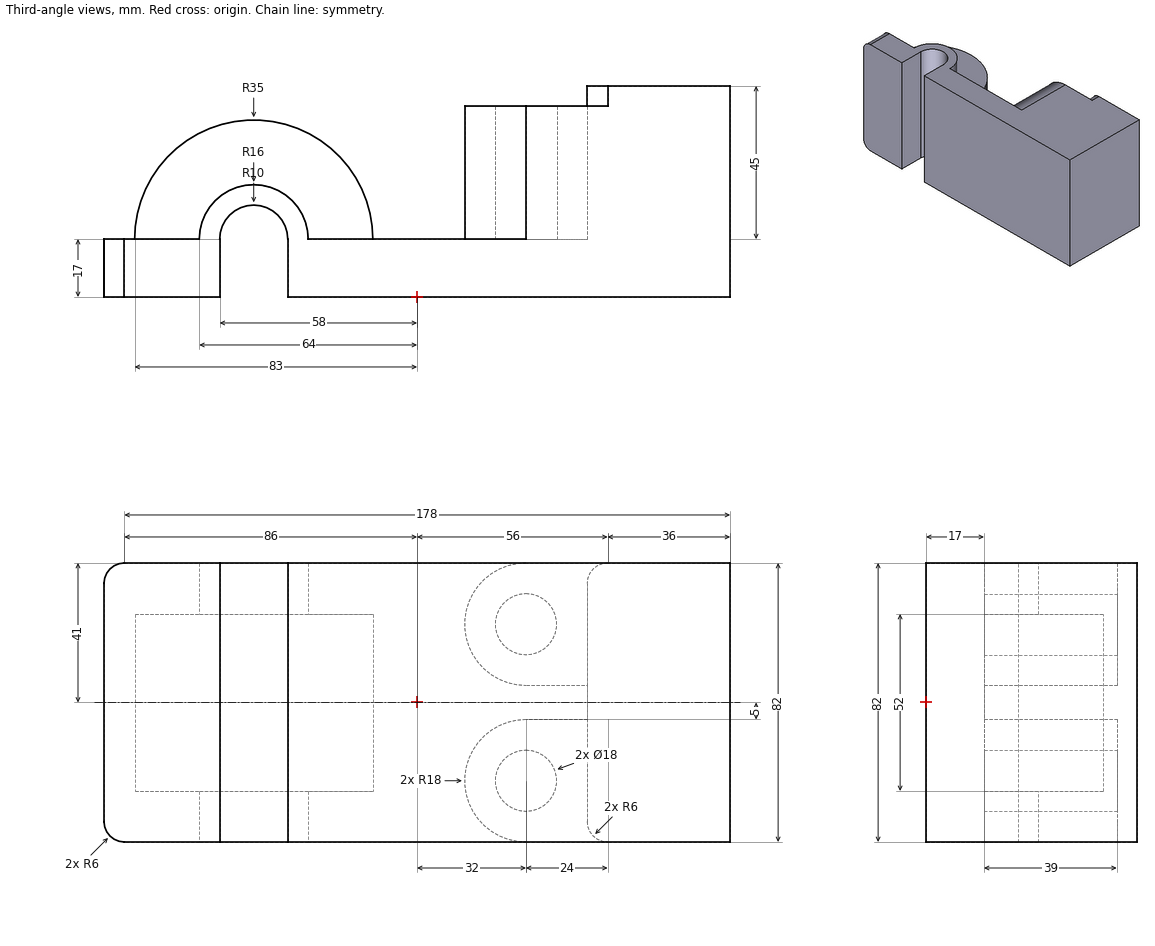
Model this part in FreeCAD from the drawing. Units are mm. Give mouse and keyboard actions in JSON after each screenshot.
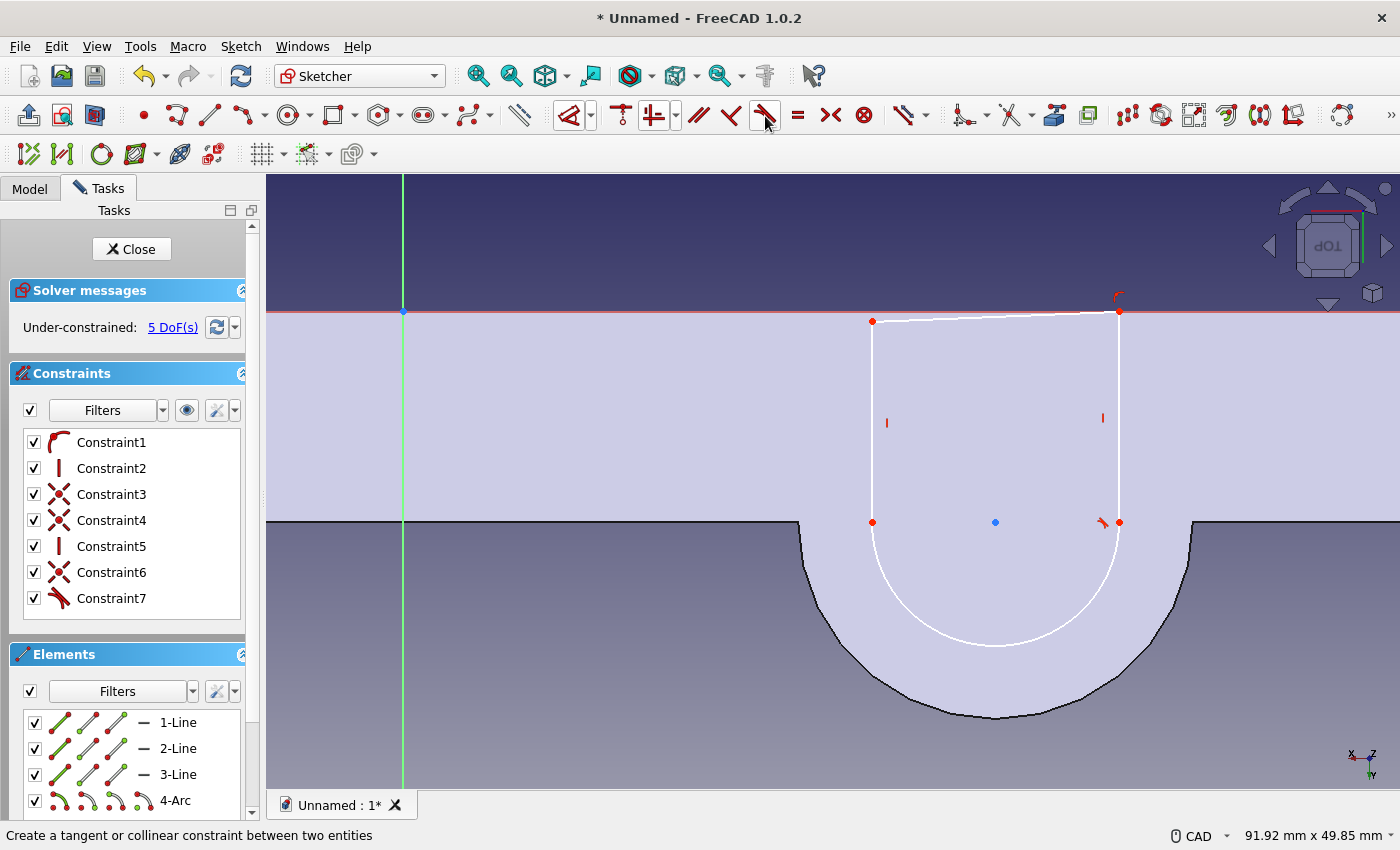
{"action": "left_click", "coordinate": [872, 382]}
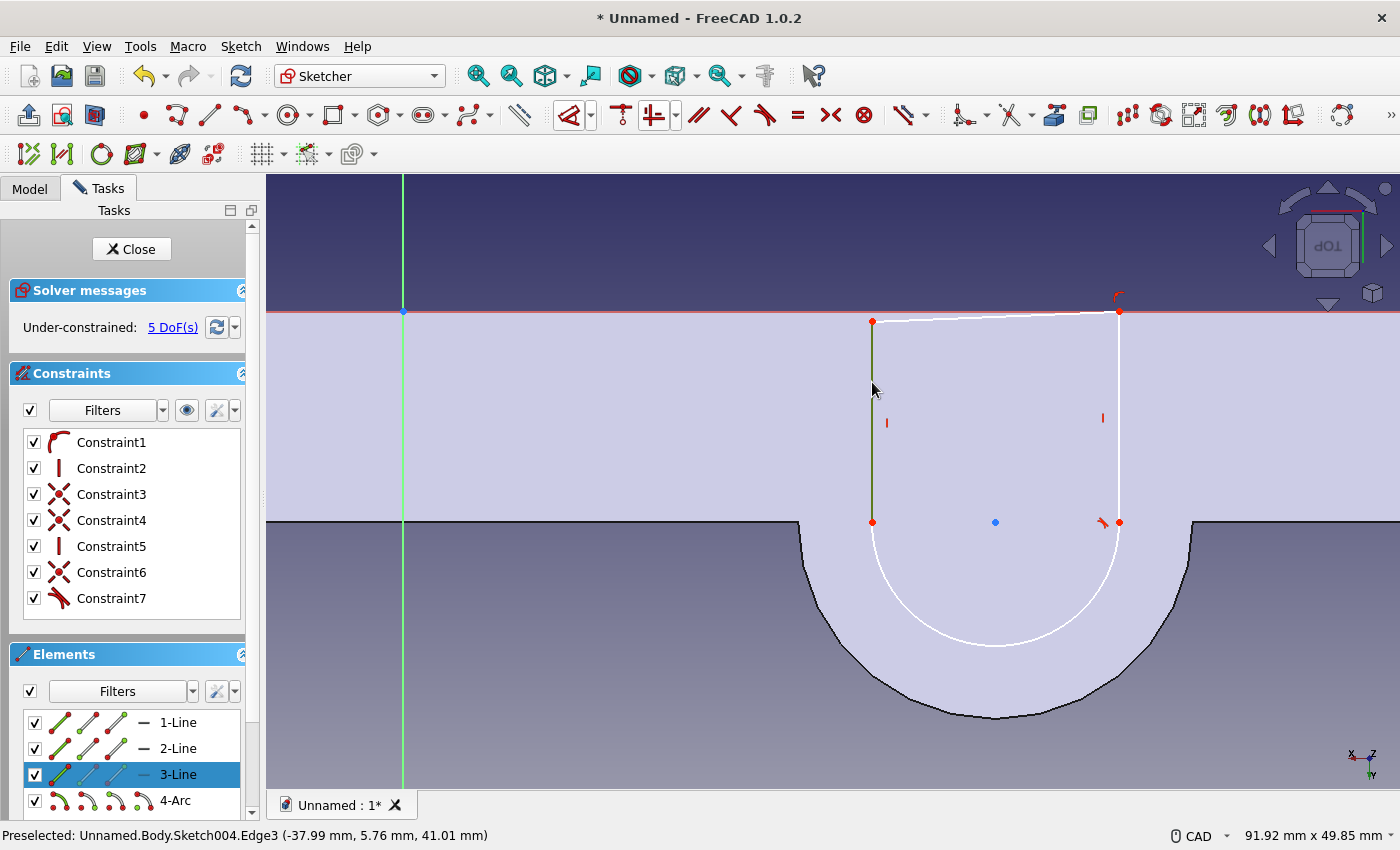
{"action": "left_click", "coordinate": [923, 623]}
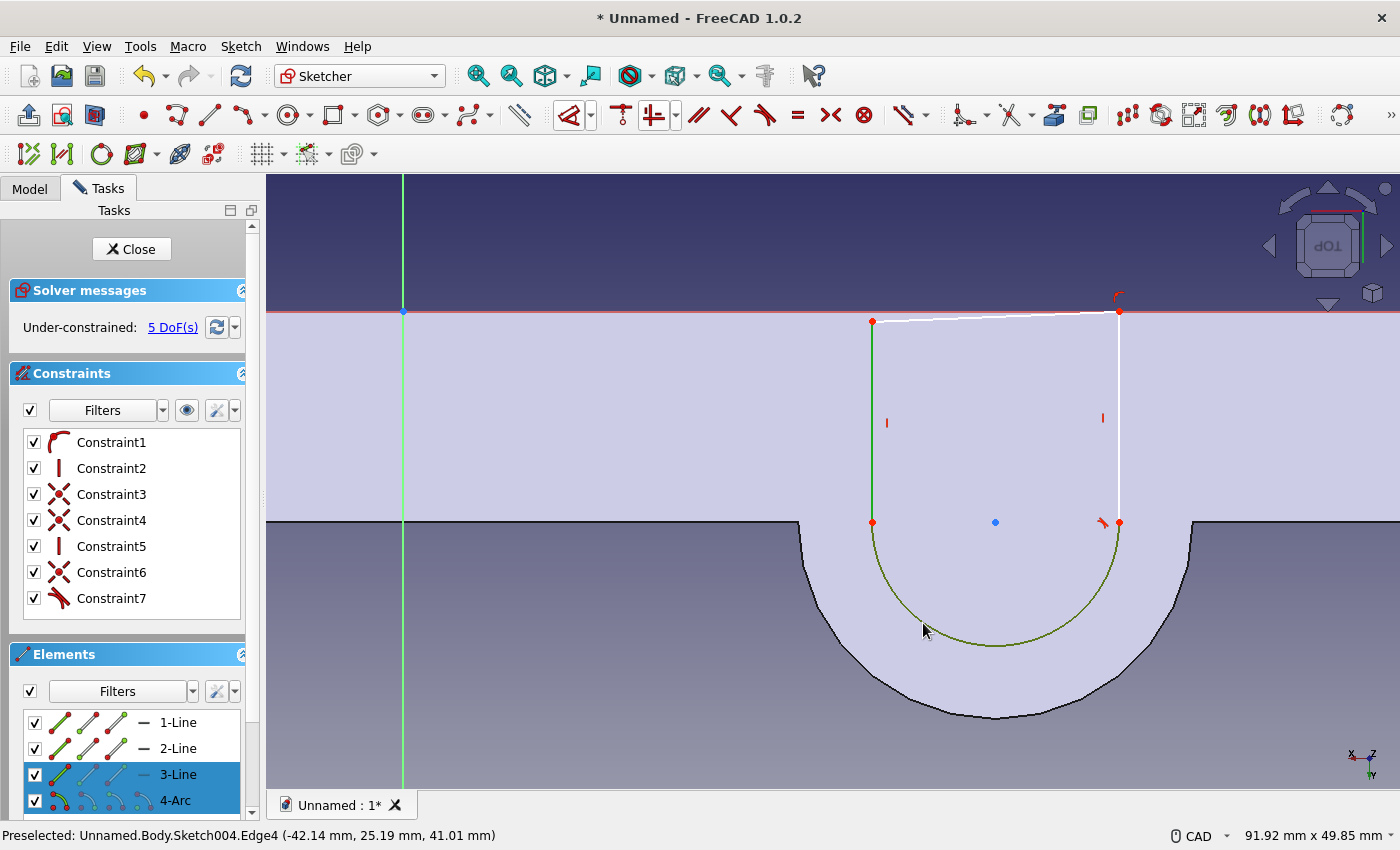
{"action": "left_click", "coordinate": [765, 116]}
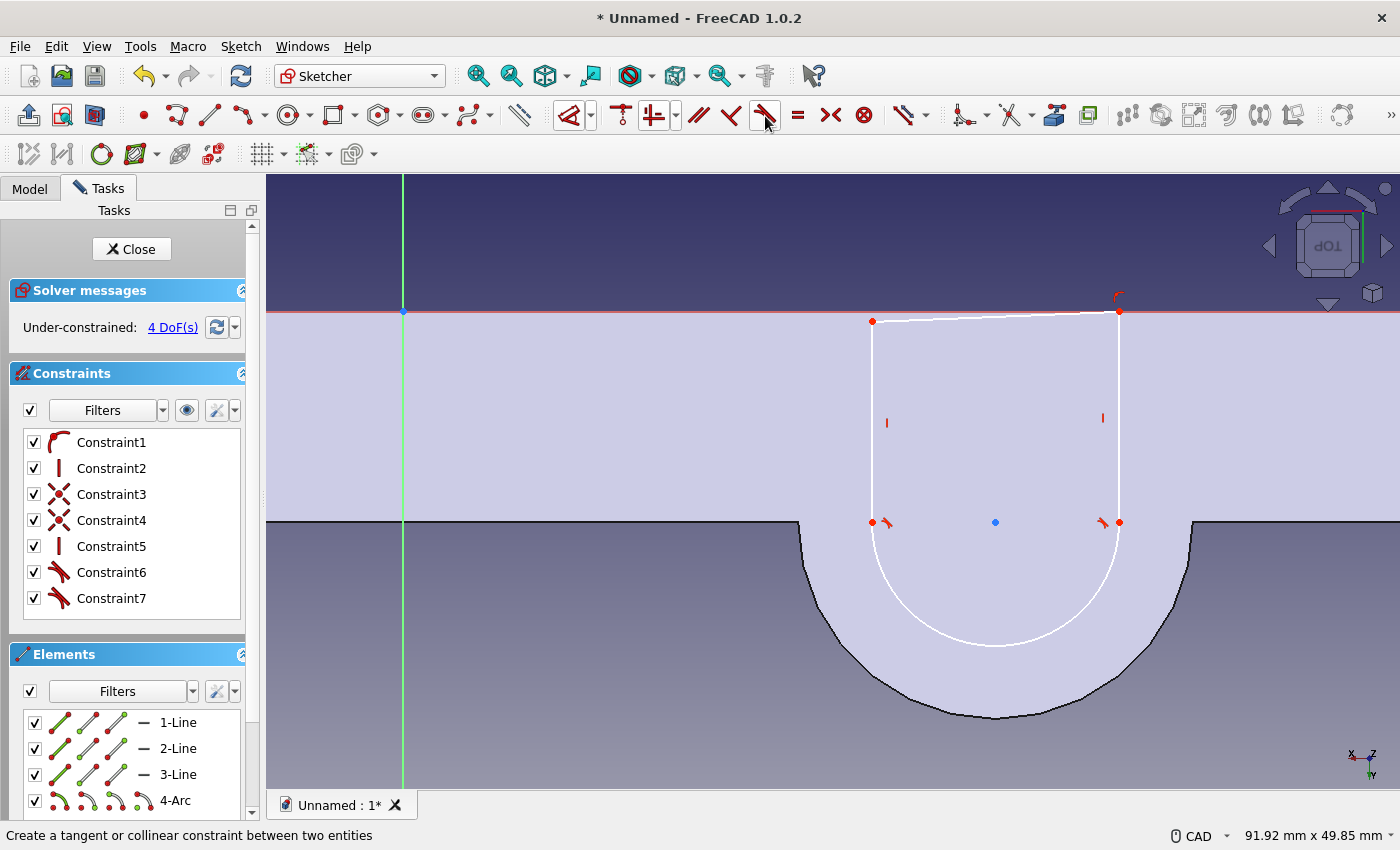
{"action": "left_click", "coordinate": [1045, 315]}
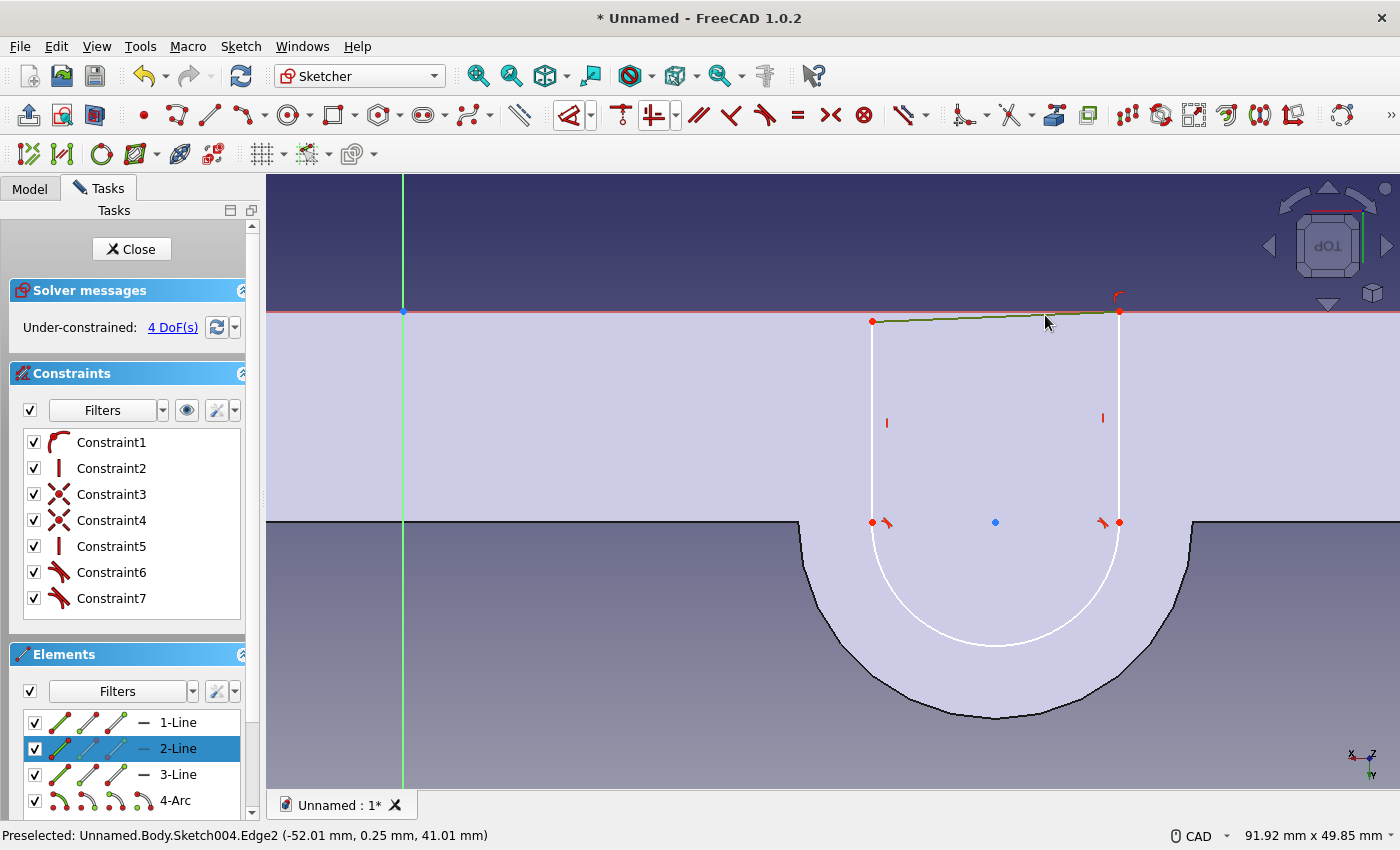
{"action": "key", "text": "h"}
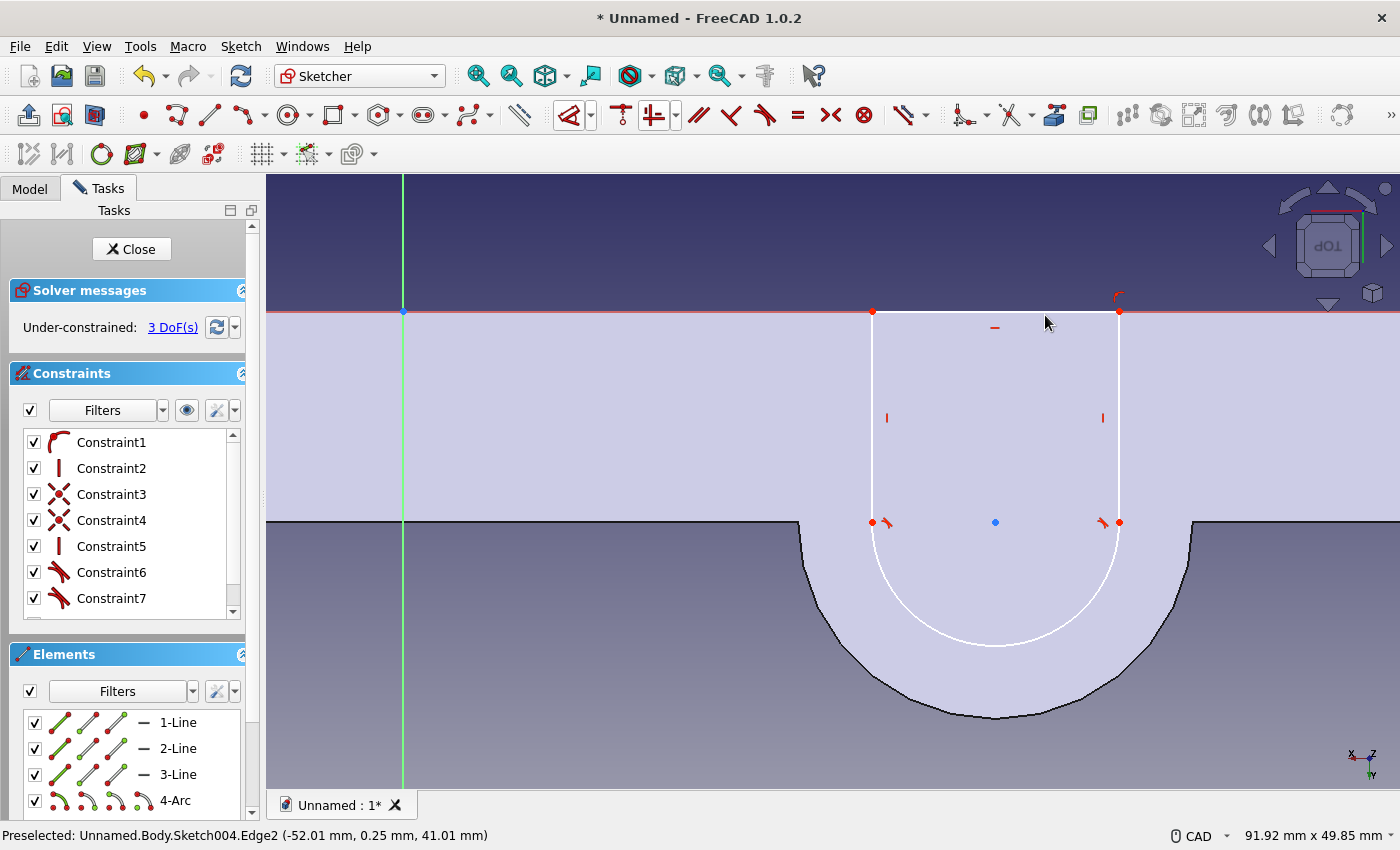
{"action": "left_click", "coordinate": [923, 622]}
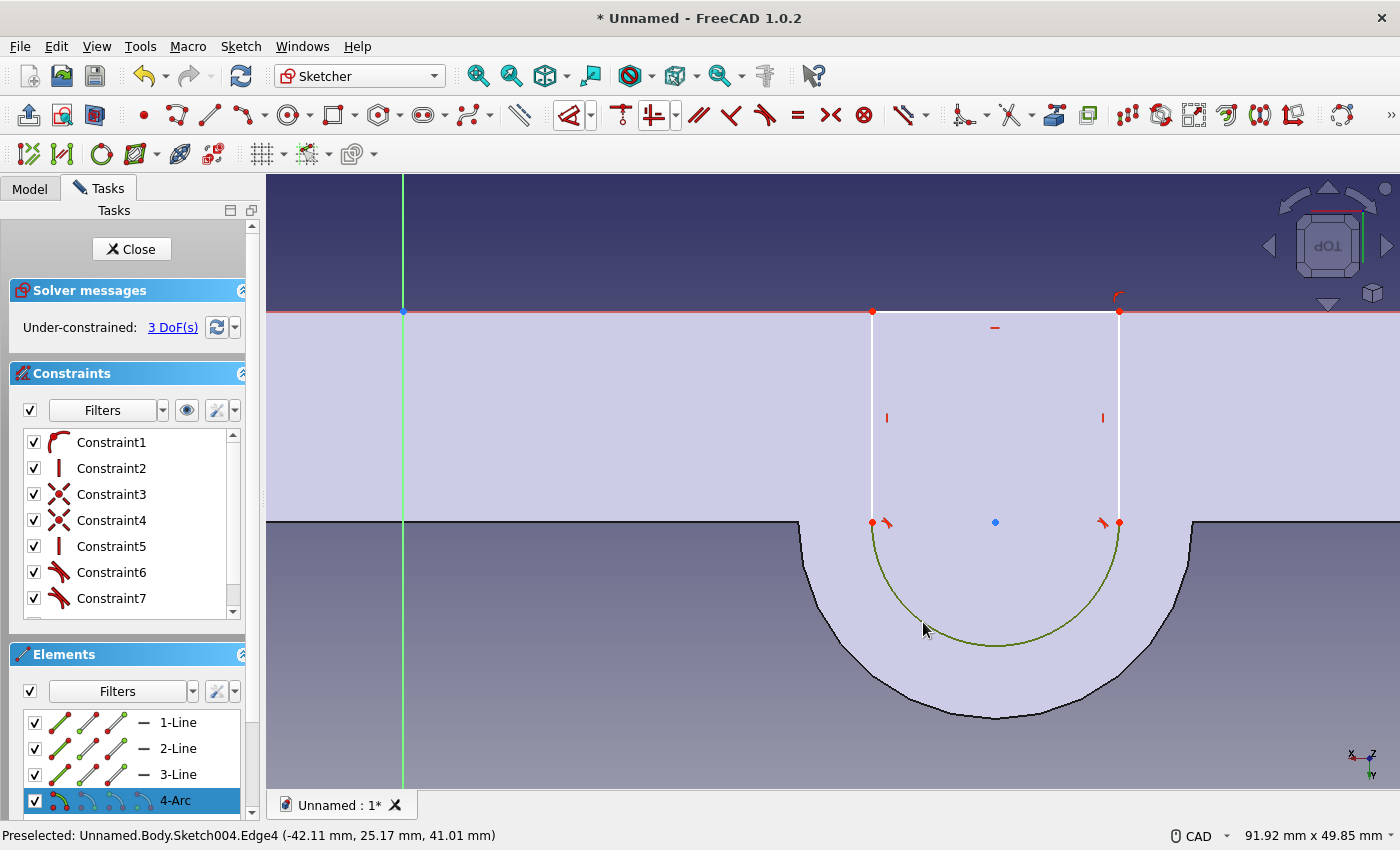
{"action": "left_click", "coordinate": [590, 116]}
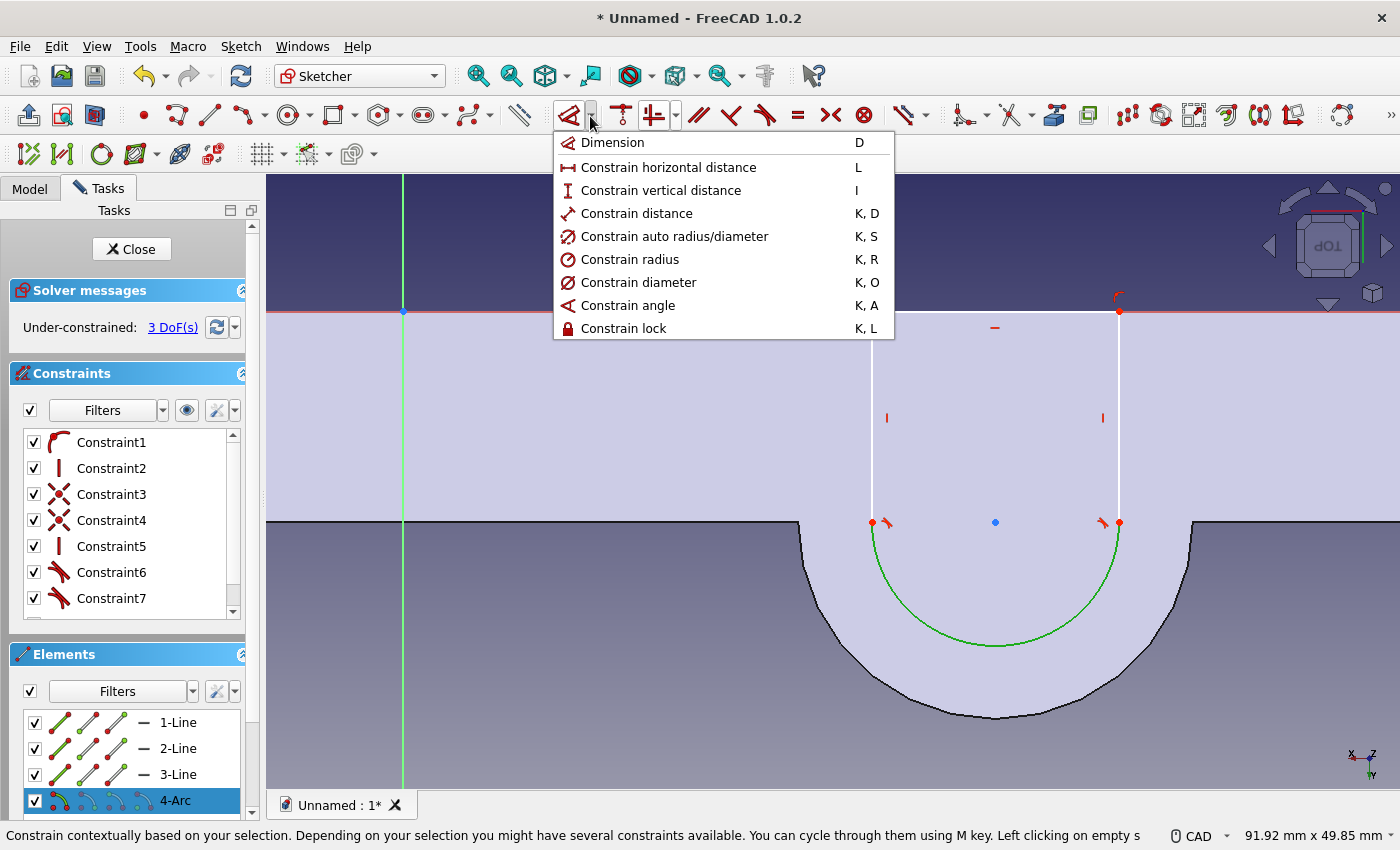
{"action": "left_click", "coordinate": [724, 260]}